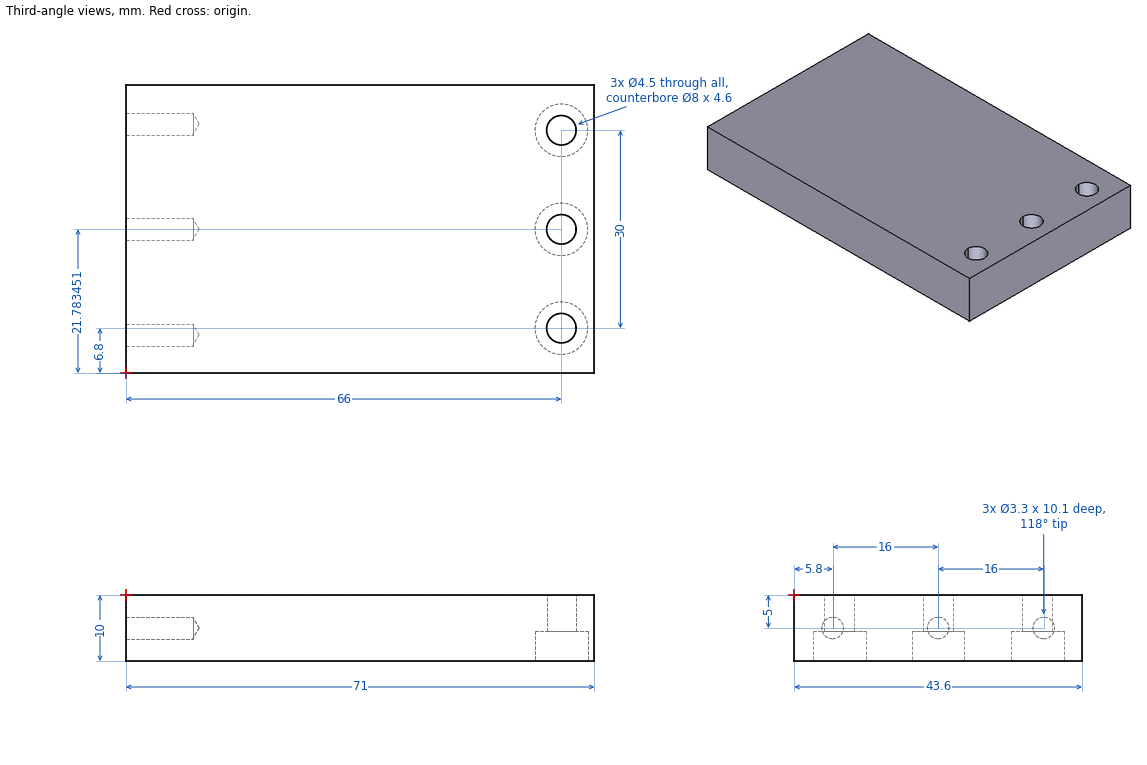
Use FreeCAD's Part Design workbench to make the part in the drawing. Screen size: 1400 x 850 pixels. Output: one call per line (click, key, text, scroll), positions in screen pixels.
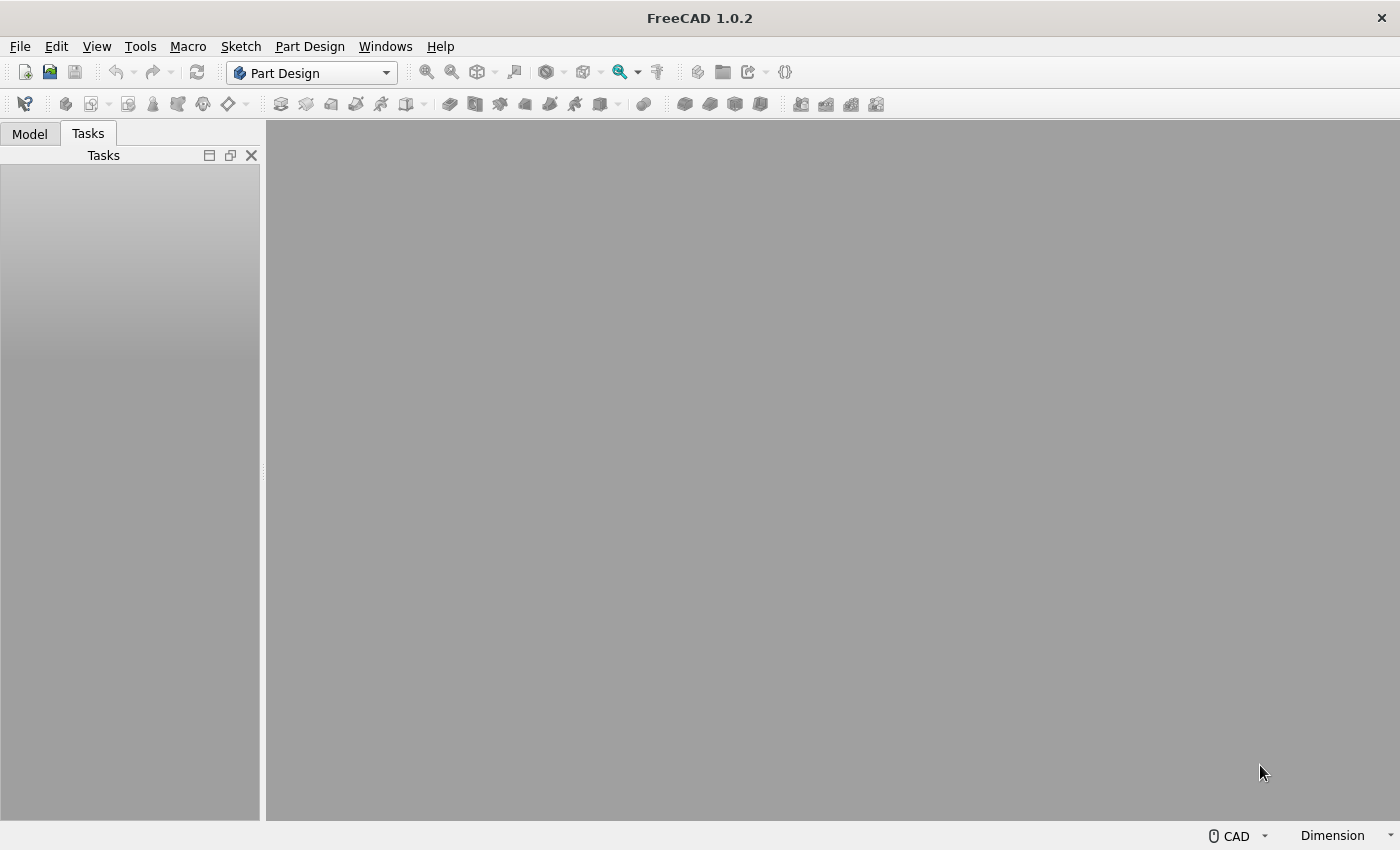
key(ctrl+n)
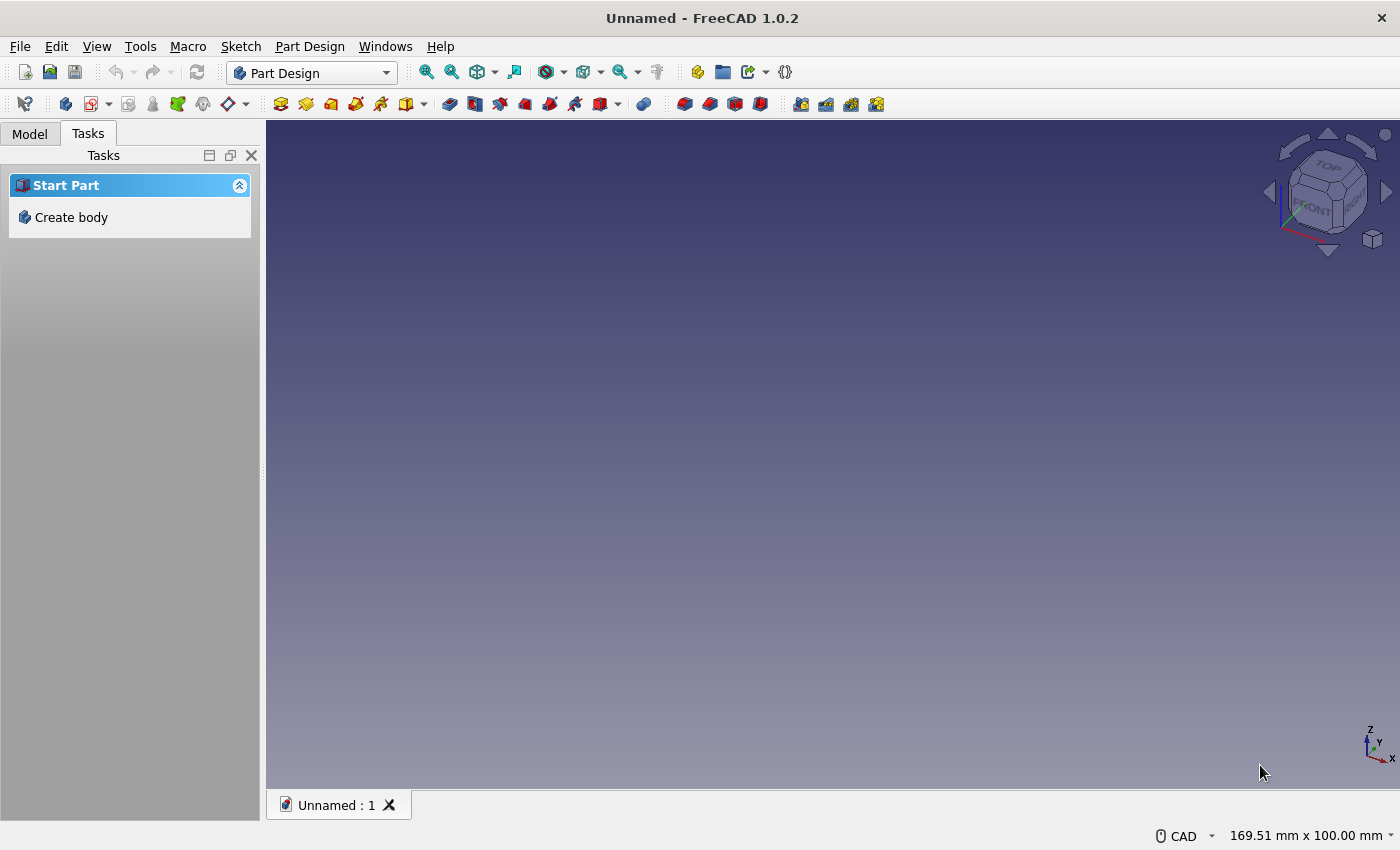
click(90, 104)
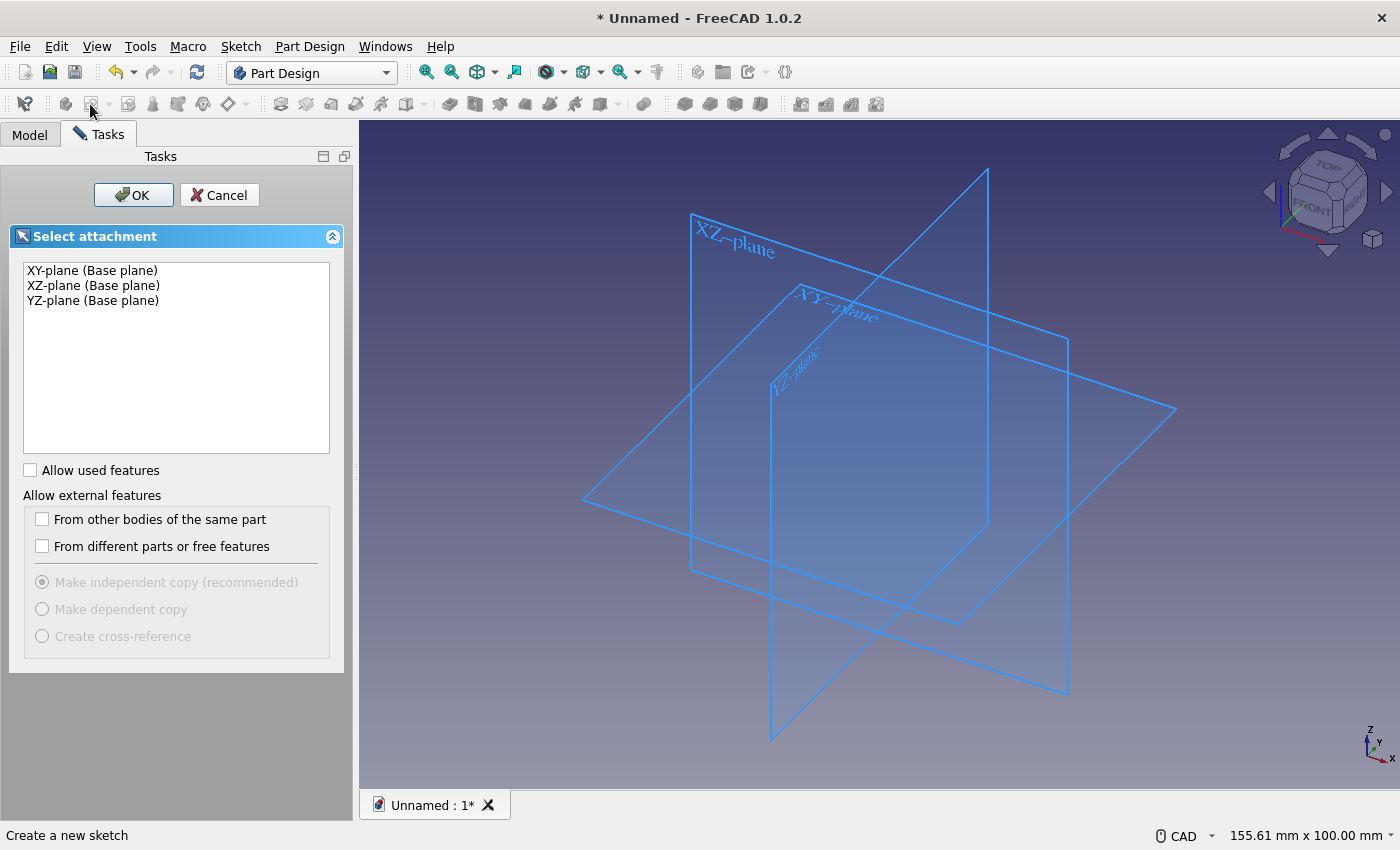
click(84, 286)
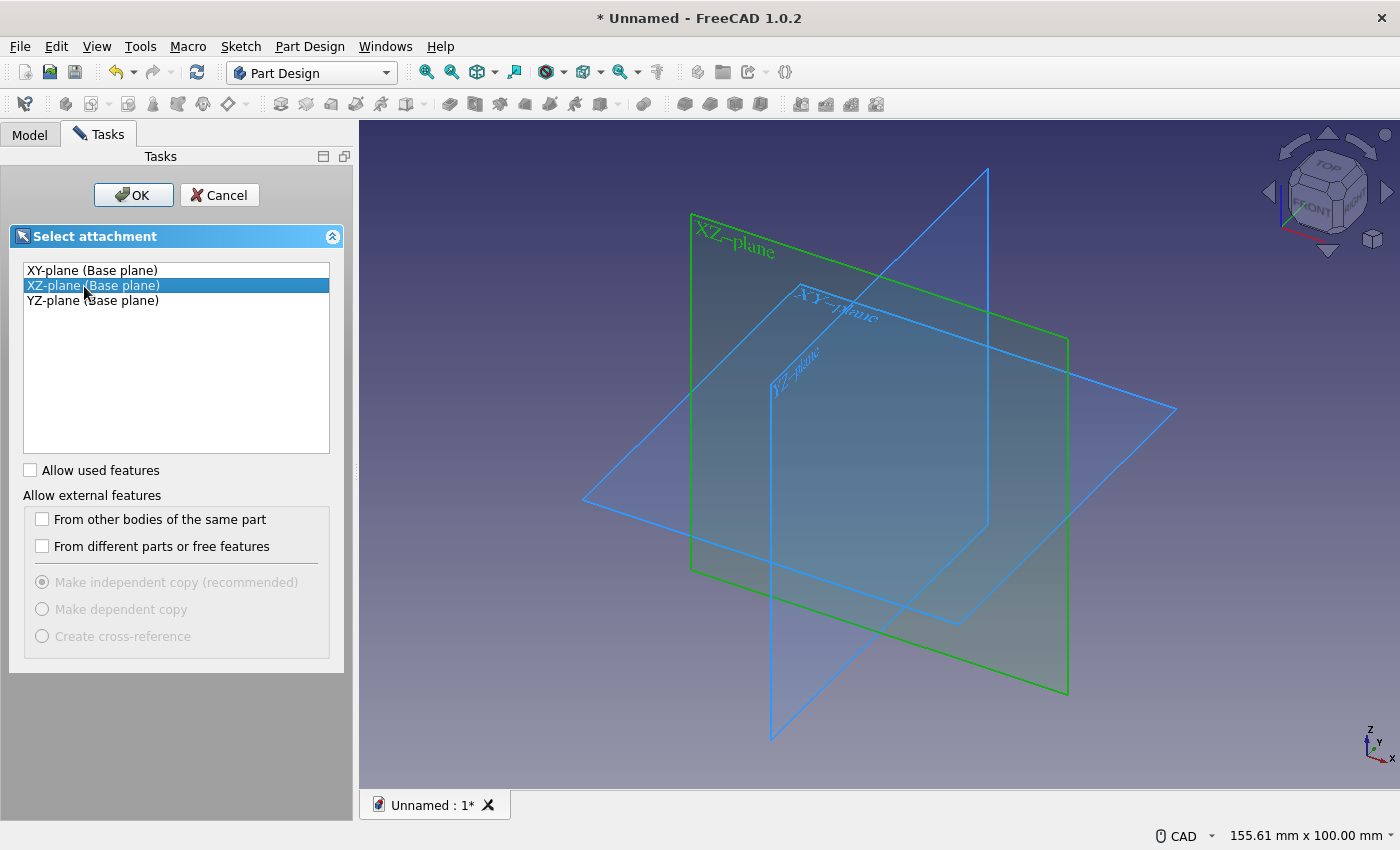
click(134, 195)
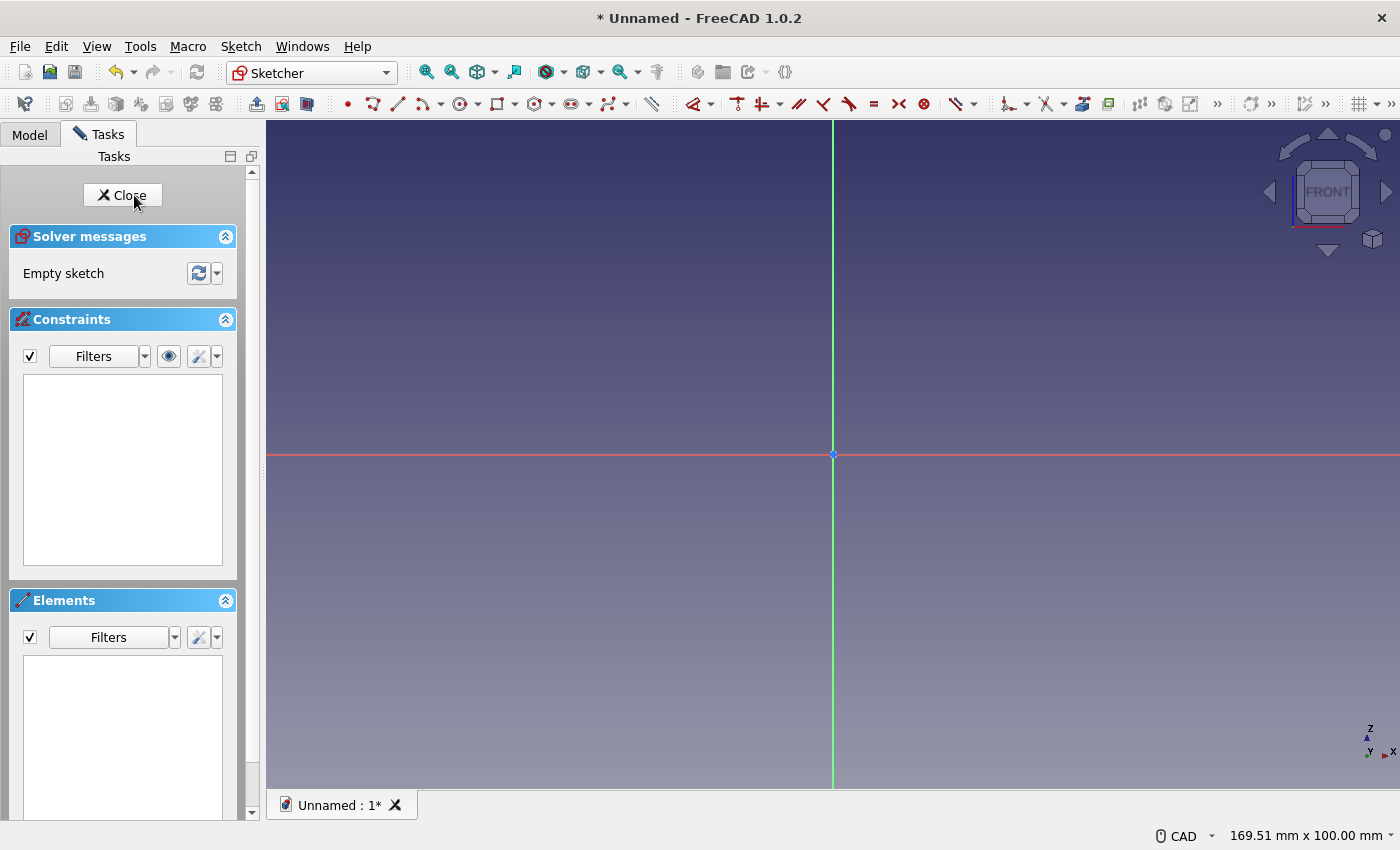
scroll(294, 303, down, 1)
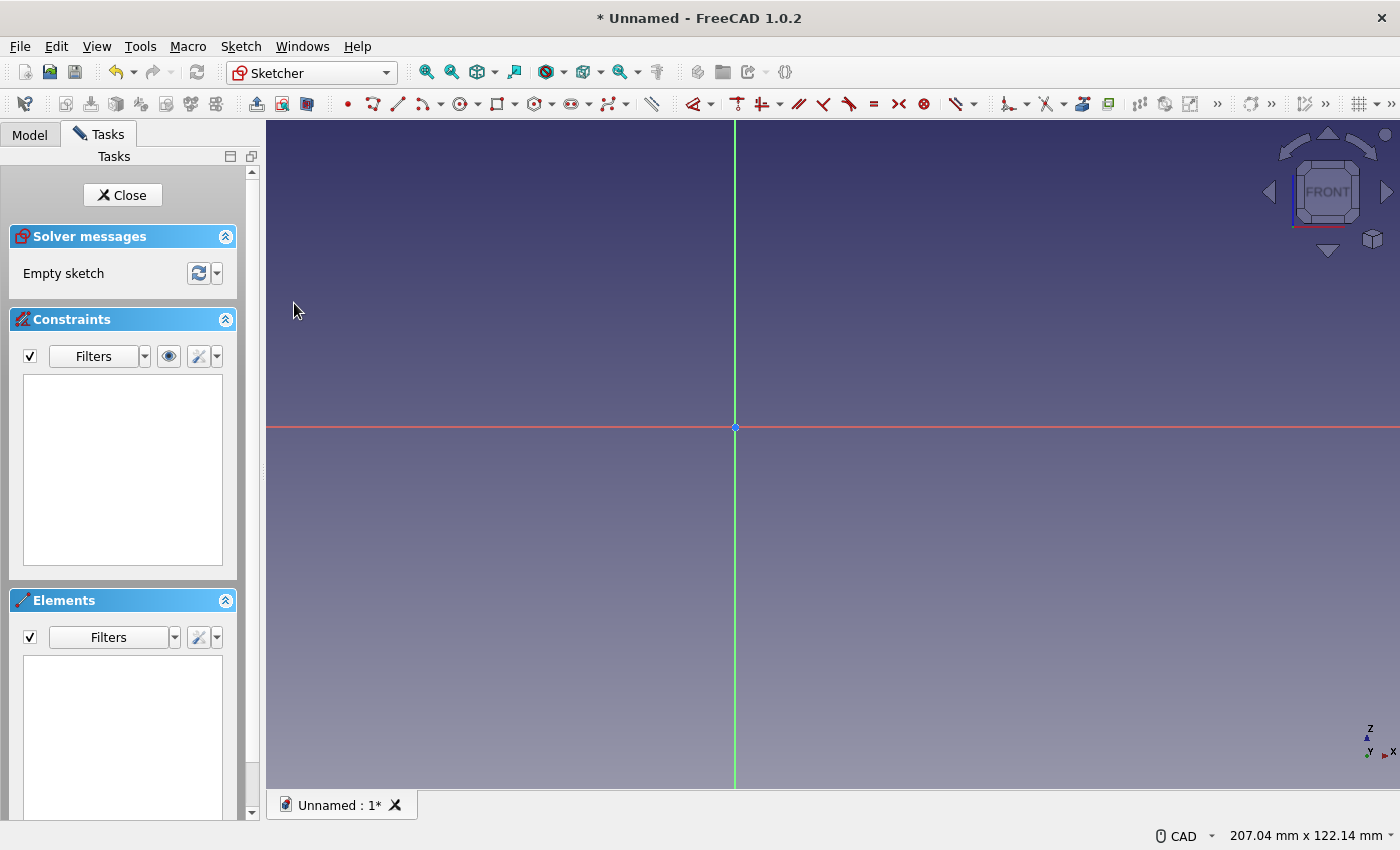
scroll(1131, 454, up, 3)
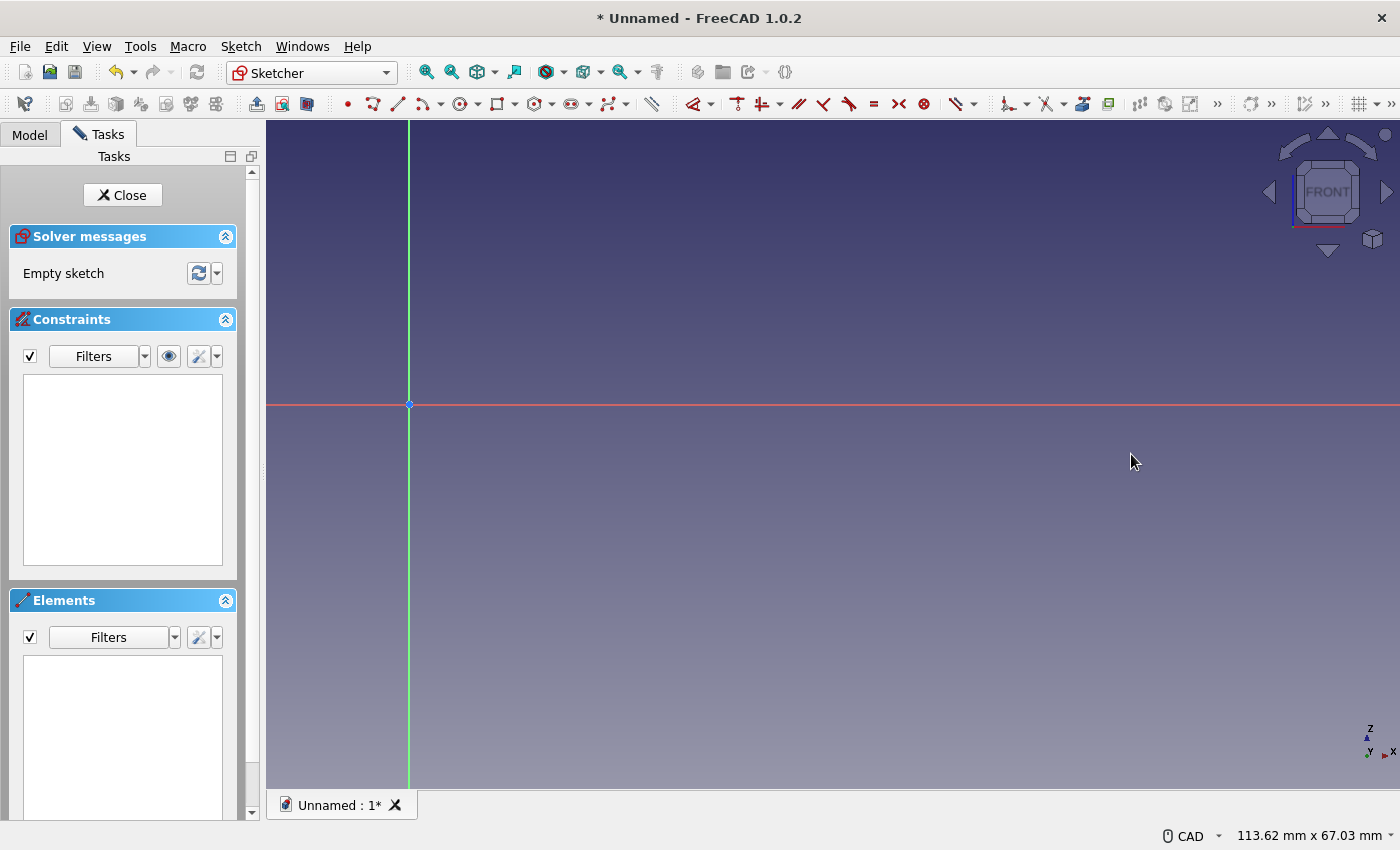
key(g)
key(r)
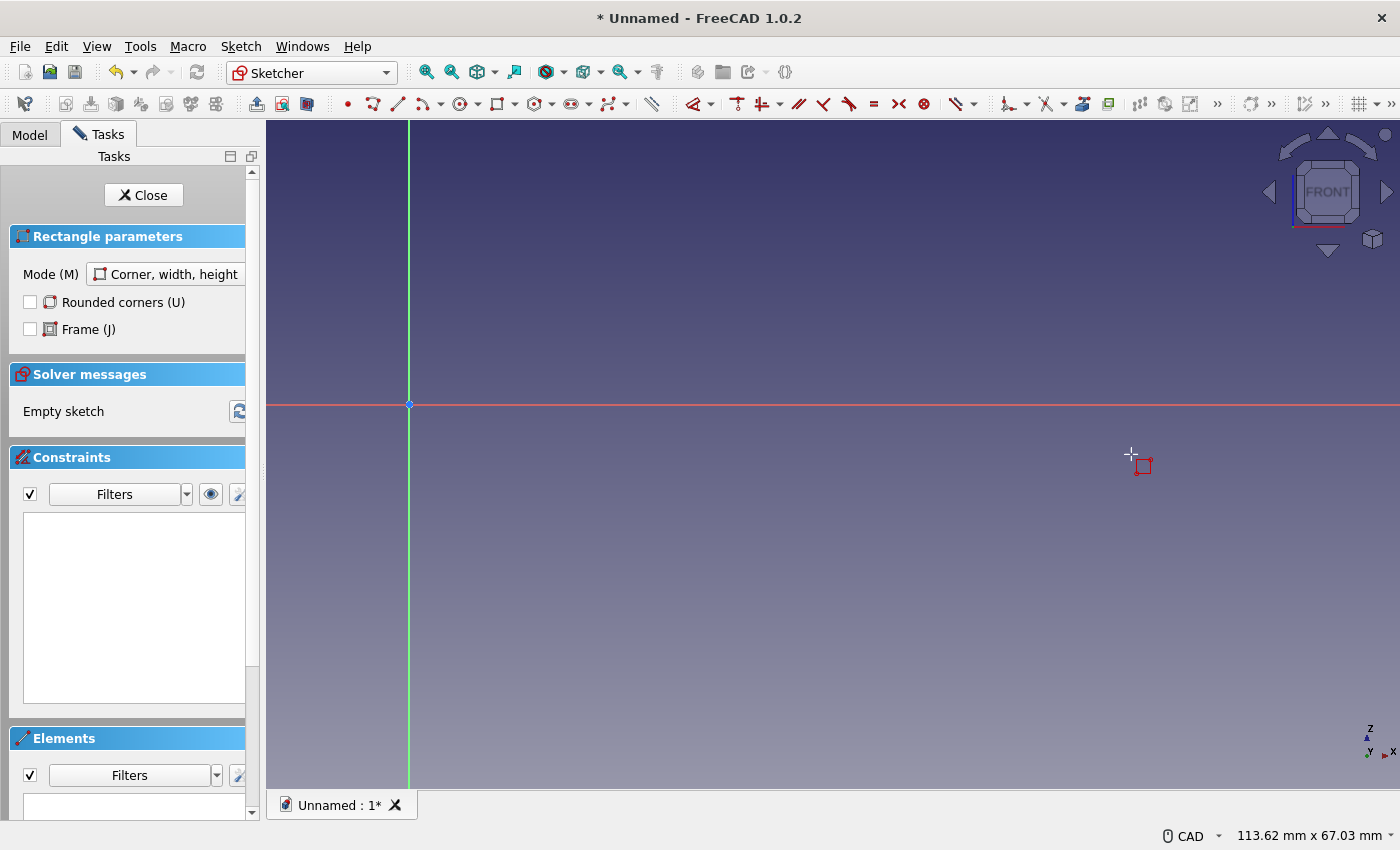
click(409, 405)
click(1118, 504)
key(Escape)